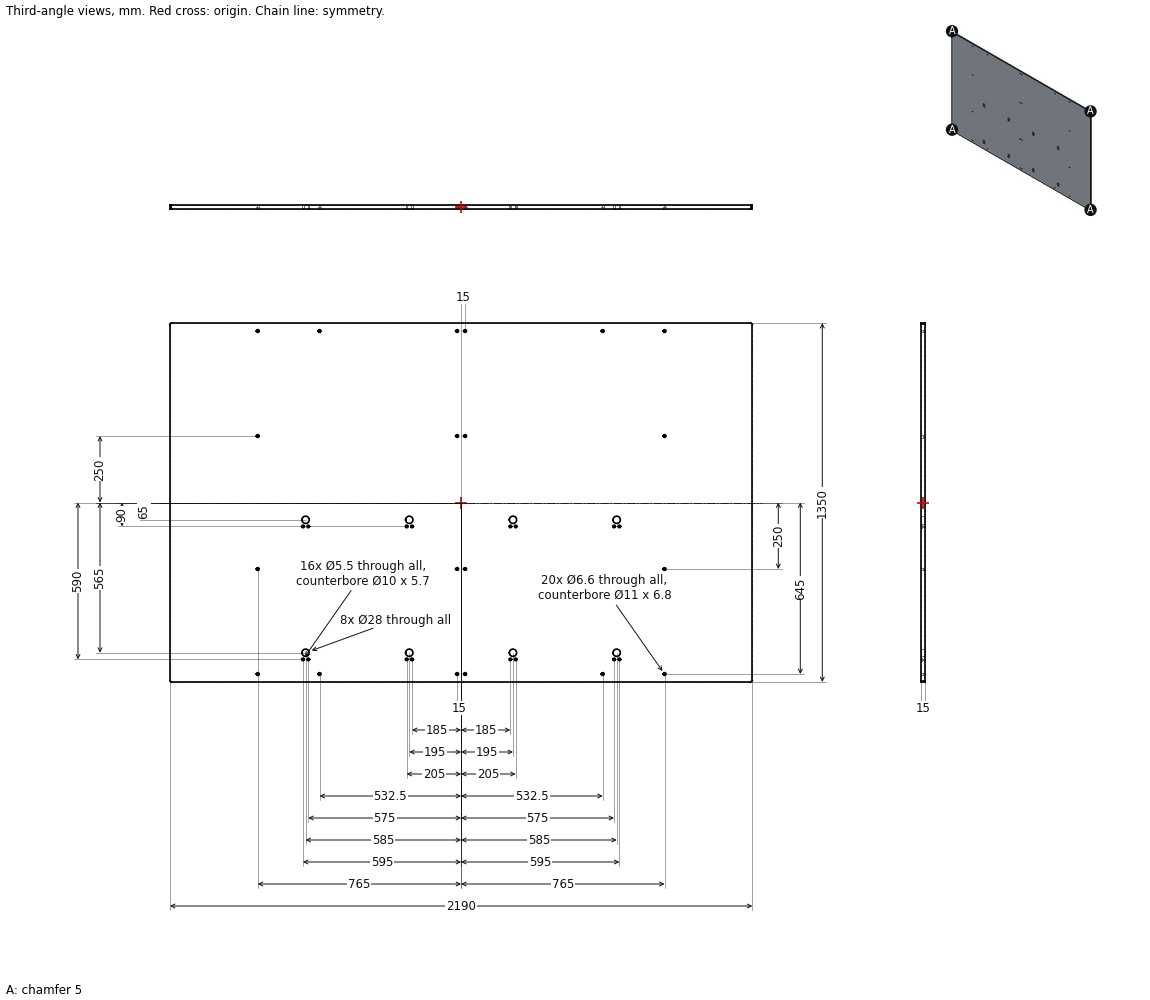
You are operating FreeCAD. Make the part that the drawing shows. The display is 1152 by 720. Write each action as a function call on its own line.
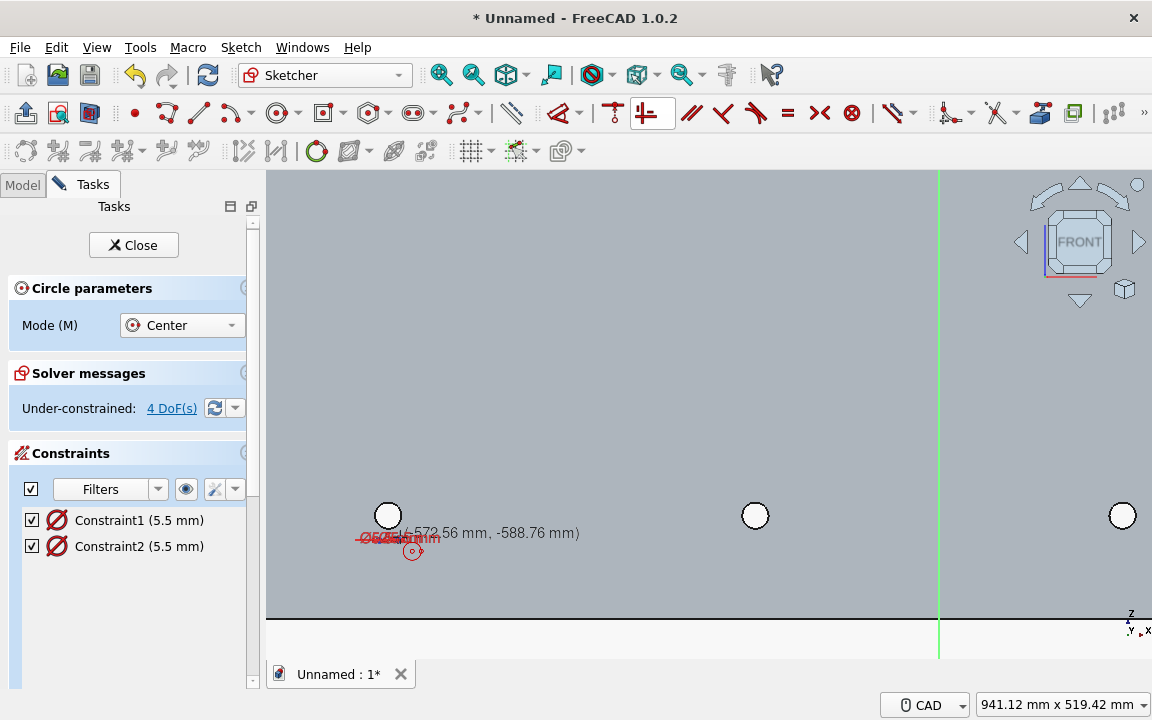
scroll(746, 539, up, 11)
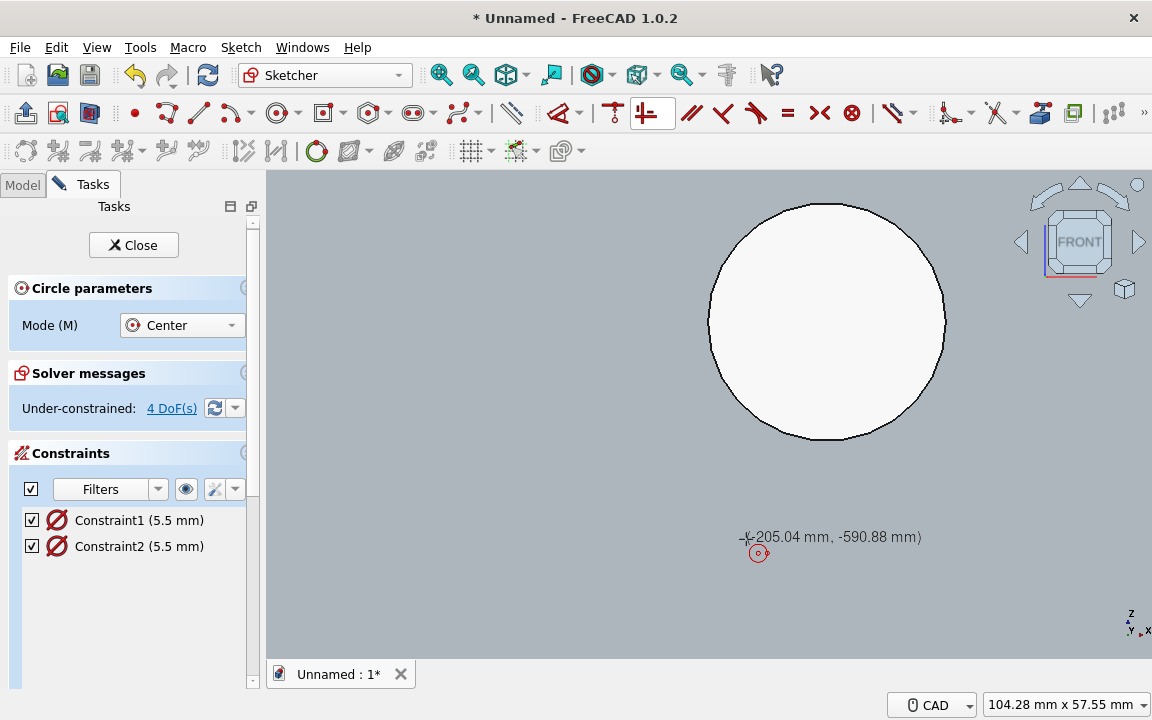
scroll(544, 539, down, 15)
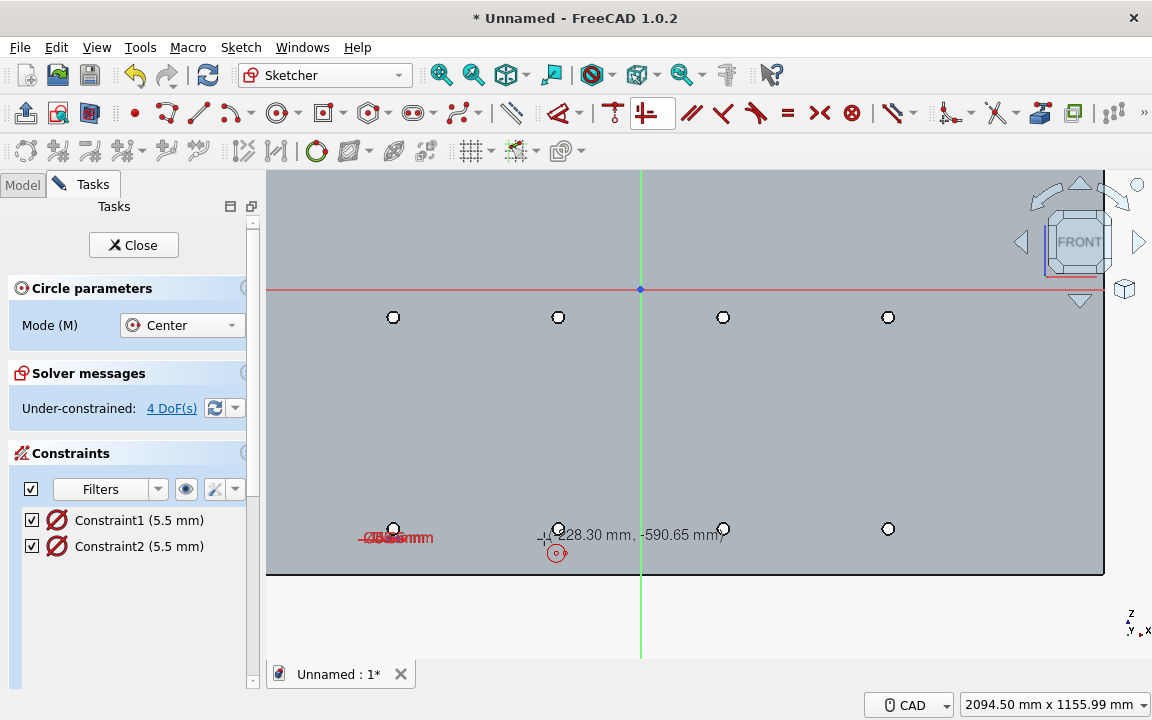
click(554, 539)
move(555, 539)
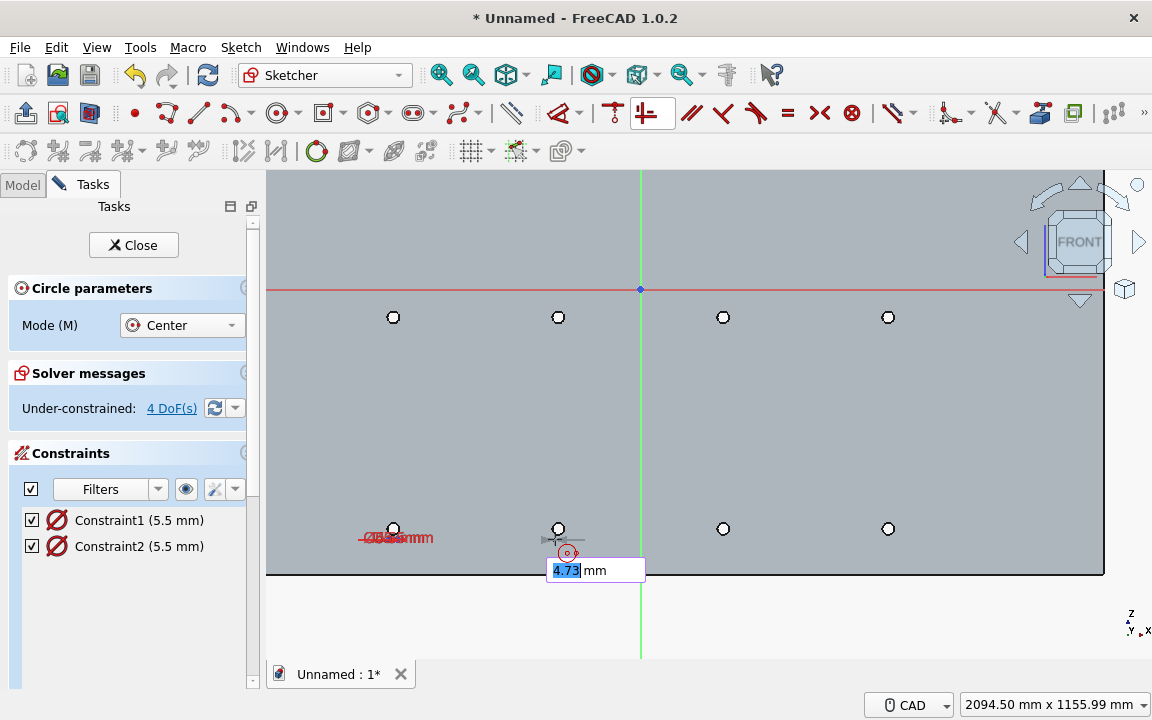
text(5.5)
key(Return)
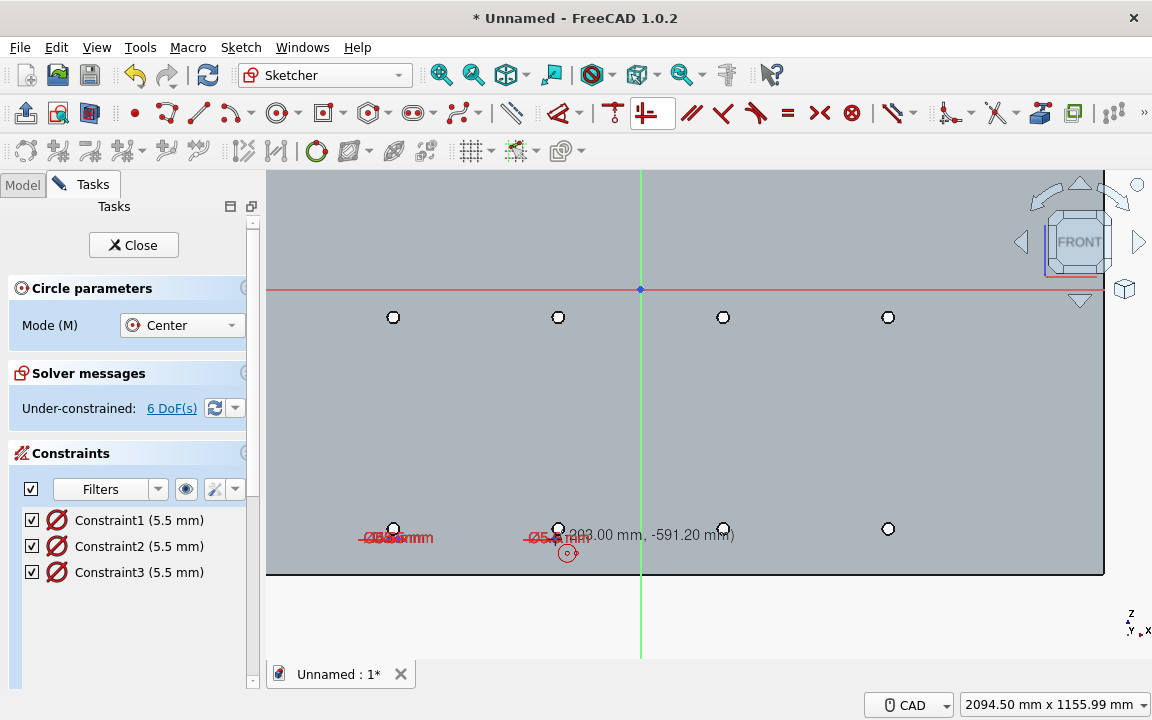
scroll(563, 539, up, 15)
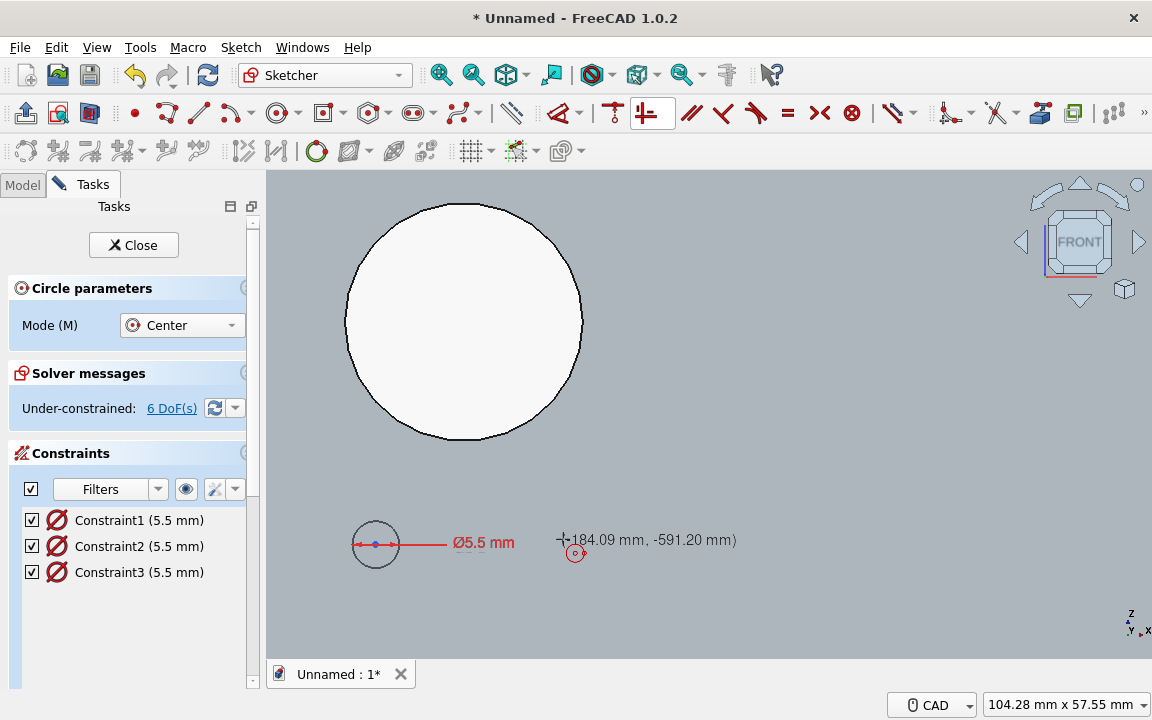
scroll(563, 539, down, 15)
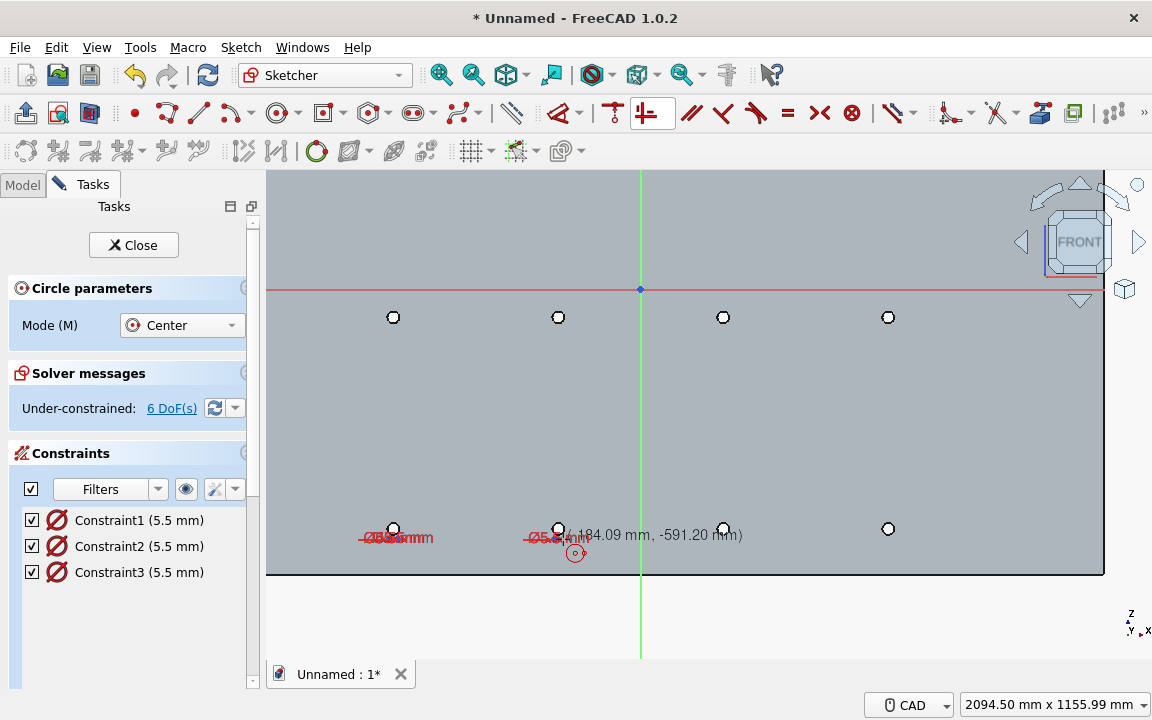
scroll(563, 539, up, 4)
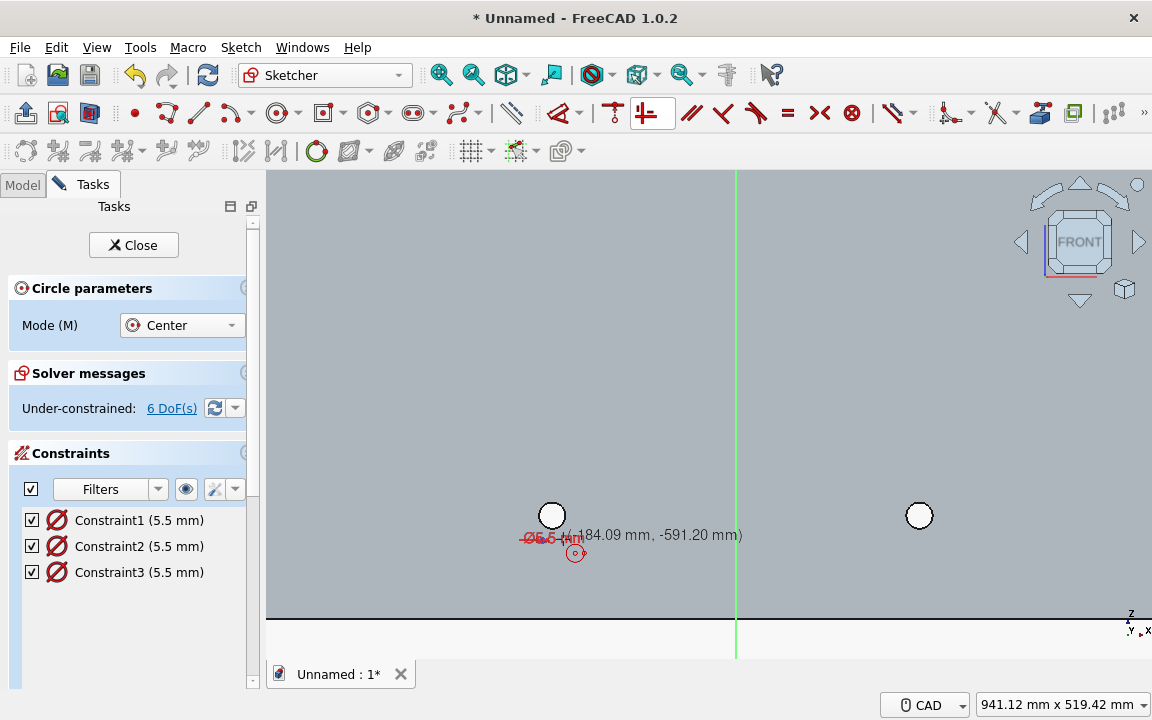
click(562, 539)
move(564, 537)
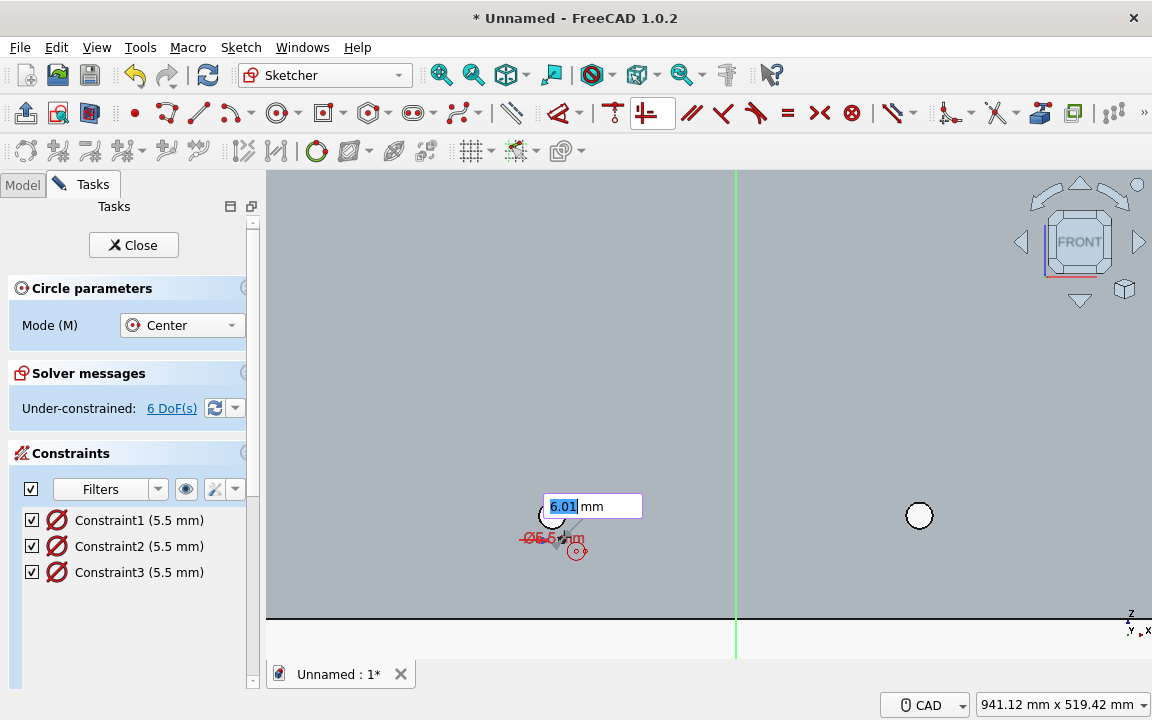
text(5.5)
key(Return)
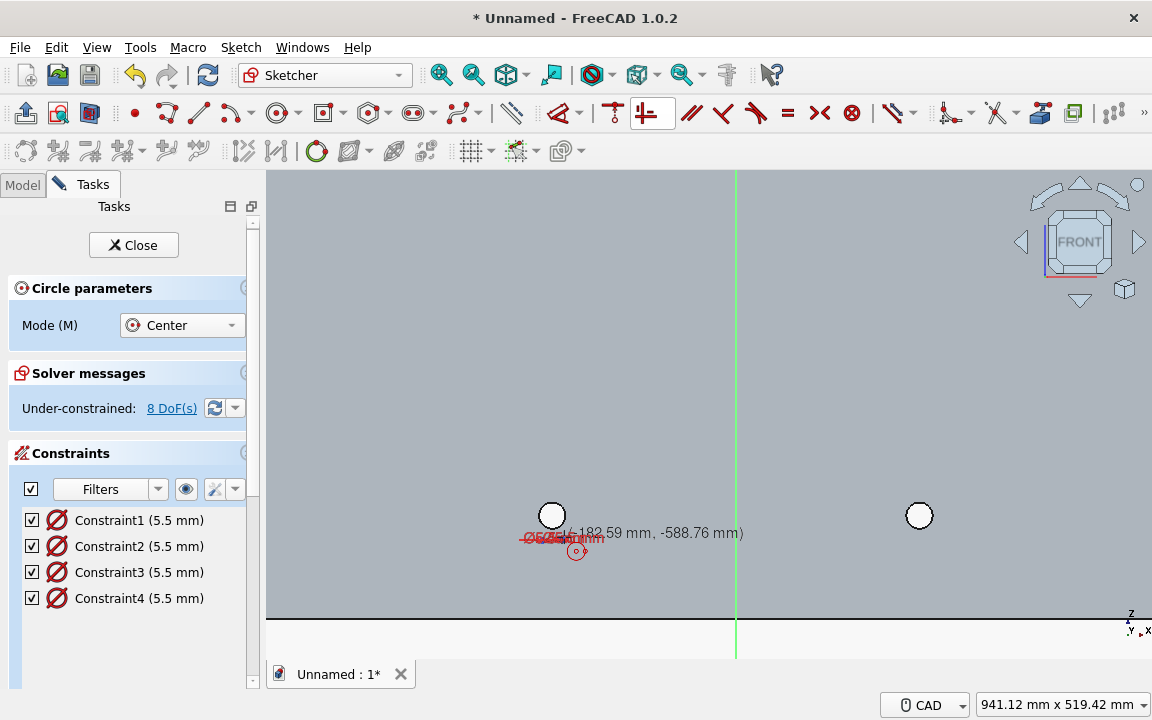
scroll(910, 539, up, 11)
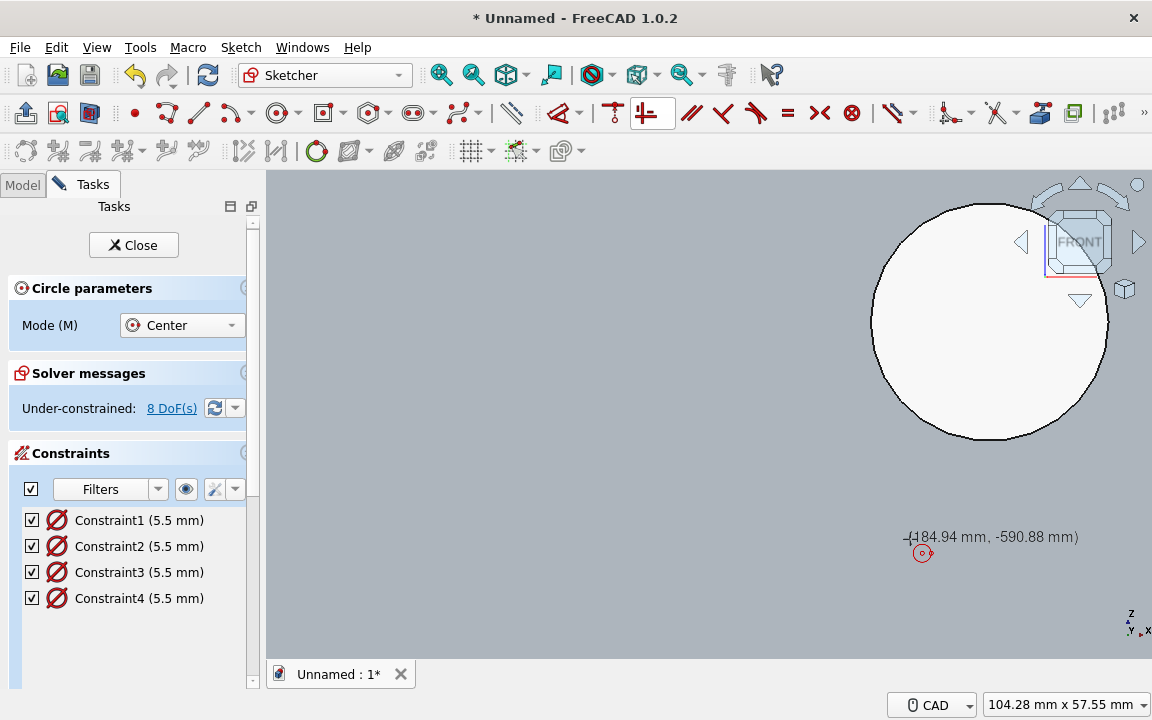
scroll(709, 539, down, 15)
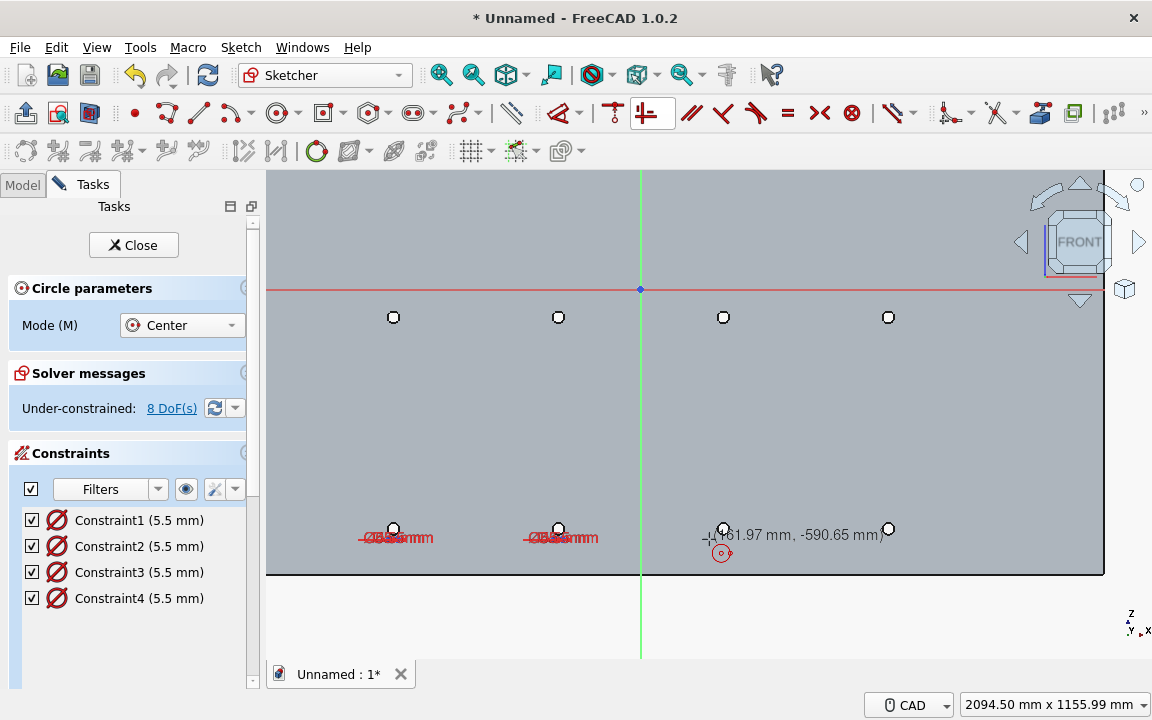
click(719, 539)
move(720, 539)